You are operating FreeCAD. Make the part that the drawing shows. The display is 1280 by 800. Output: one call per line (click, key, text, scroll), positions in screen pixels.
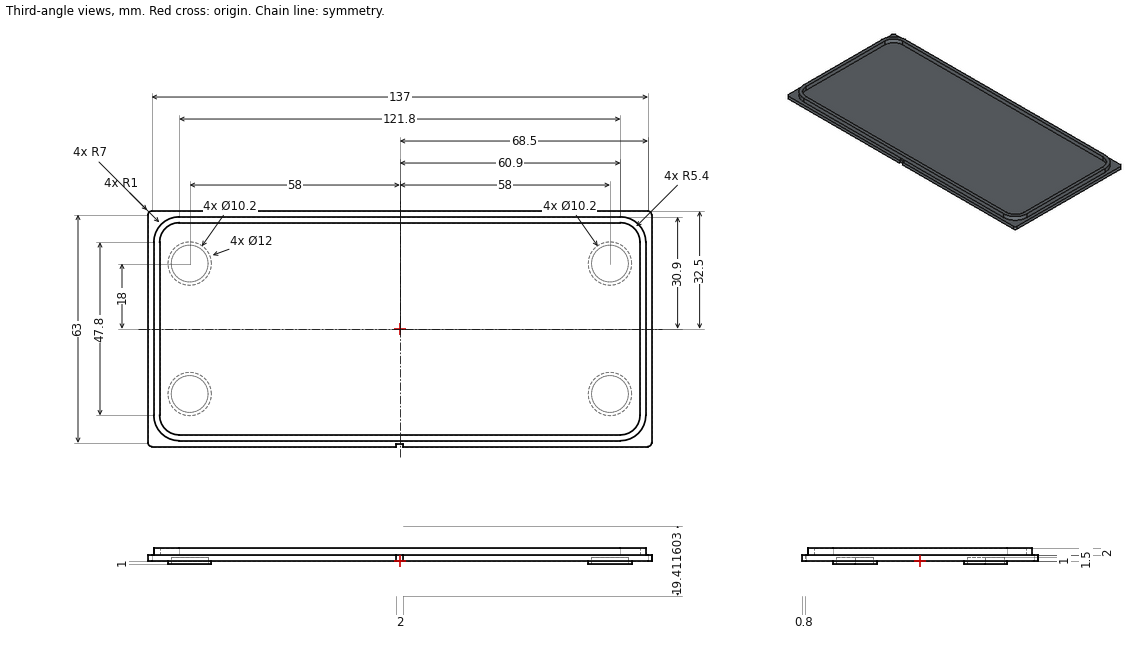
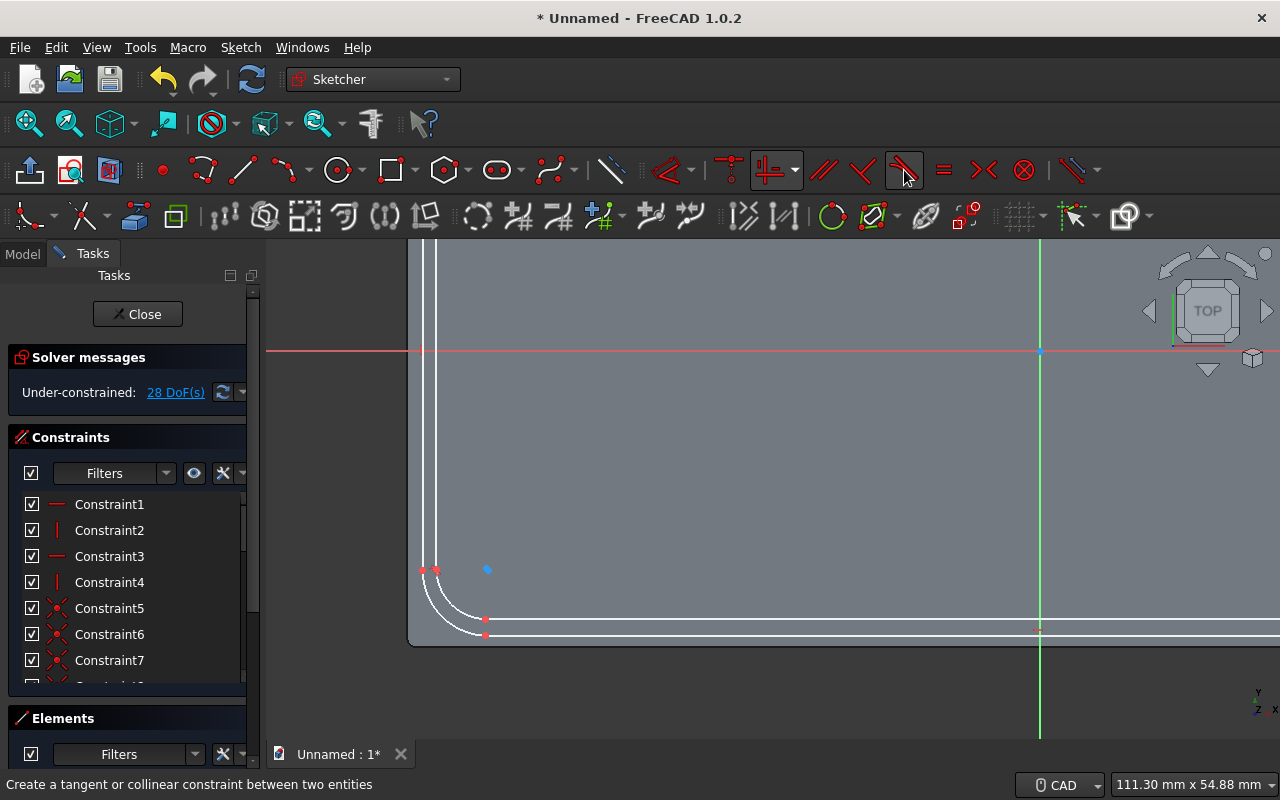
click(818, 636)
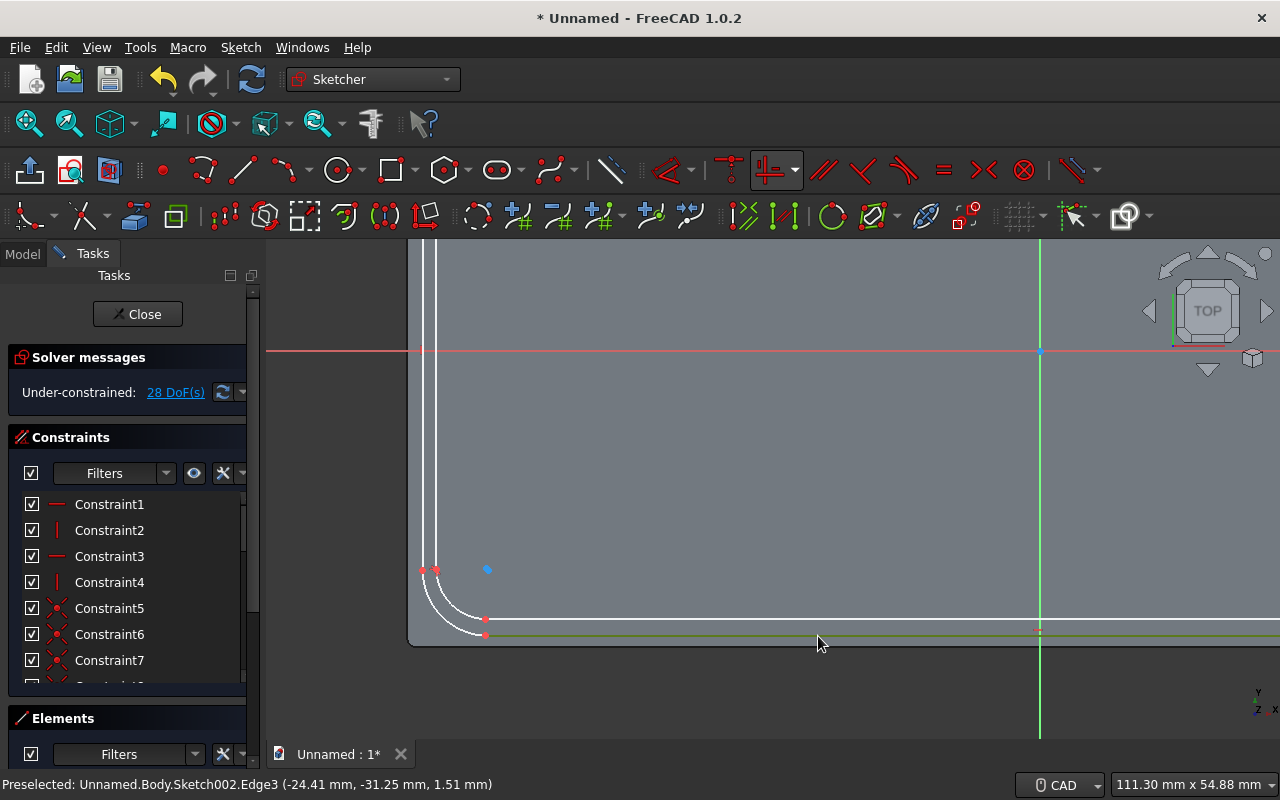
click(429, 599)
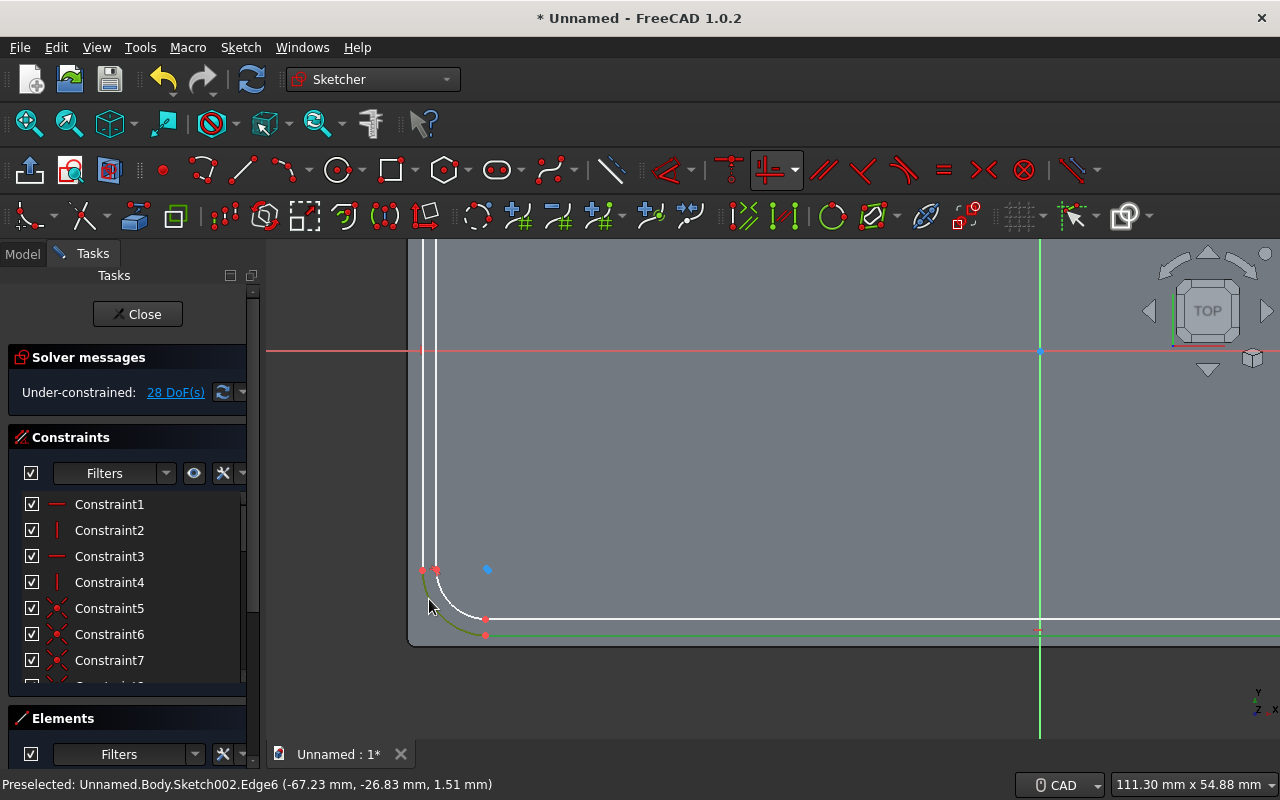
click(904, 170)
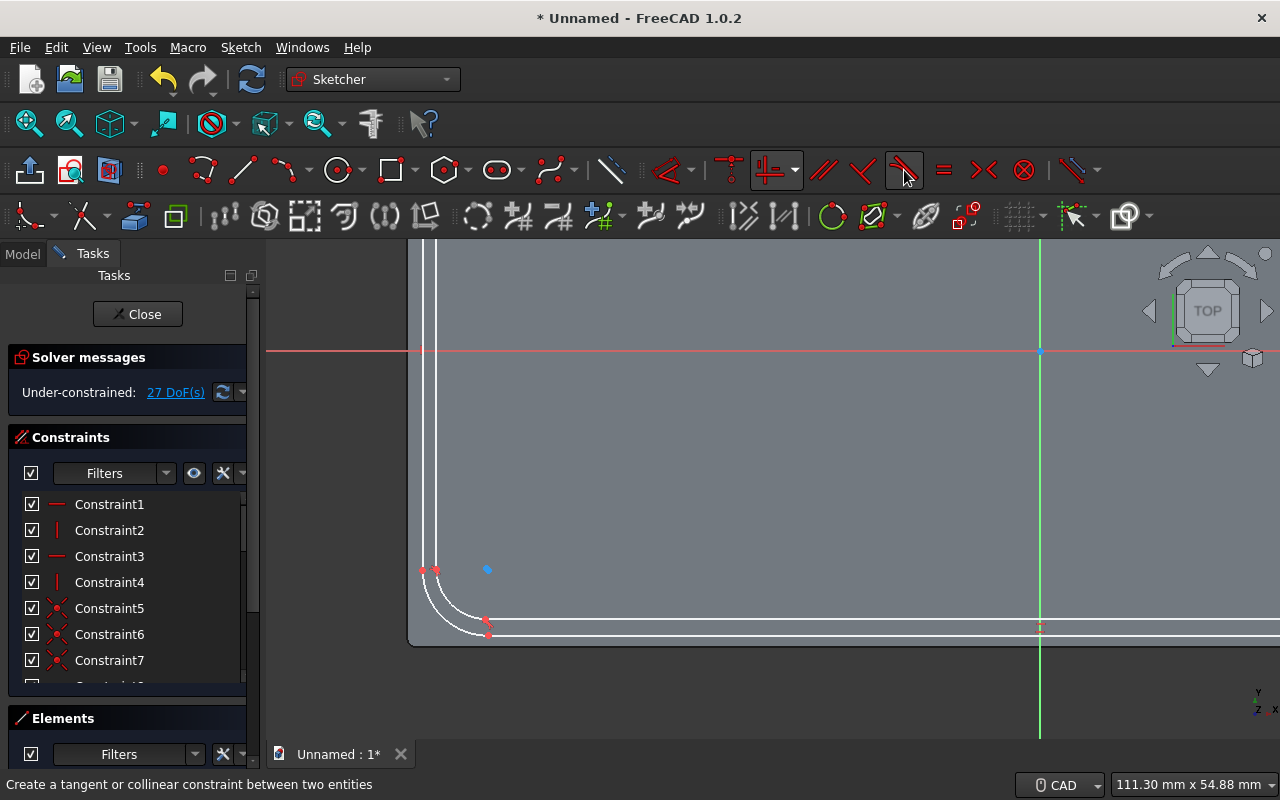
click(821, 636)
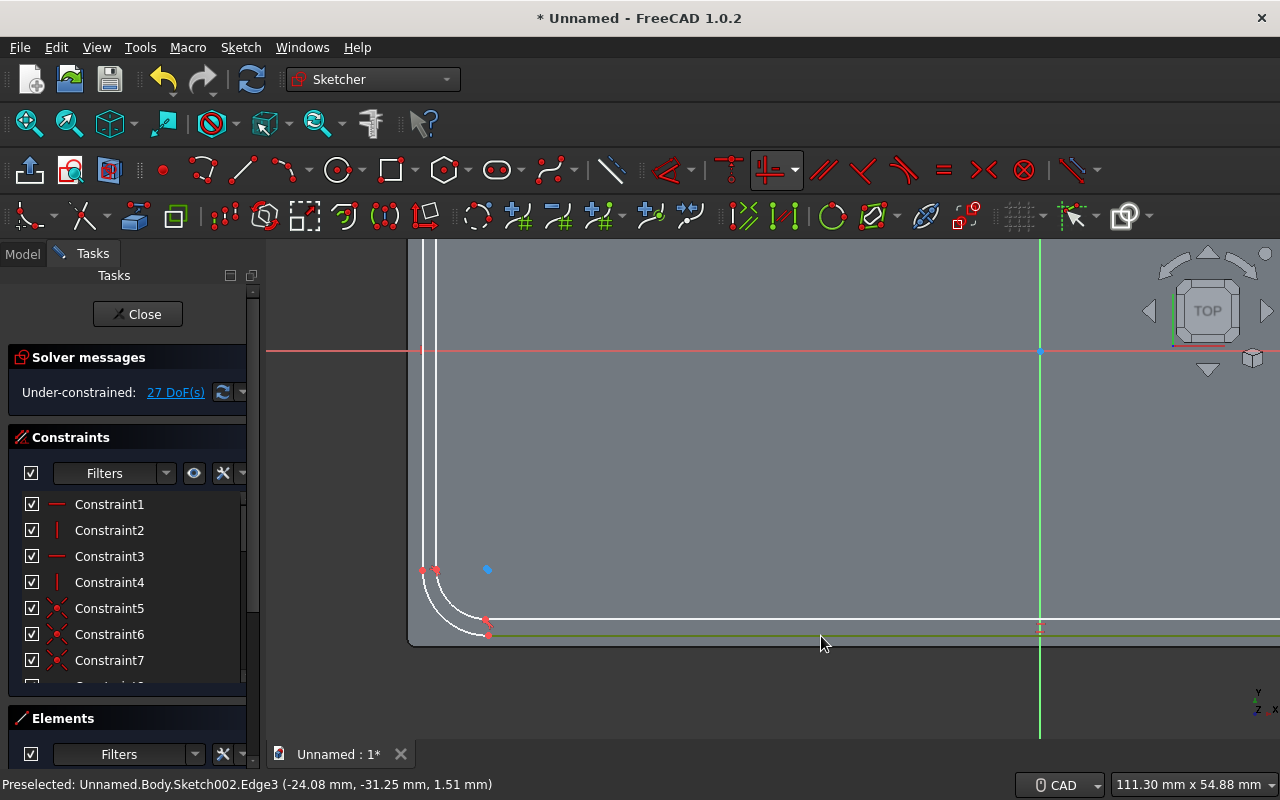
scroll(430, 602, down, 4)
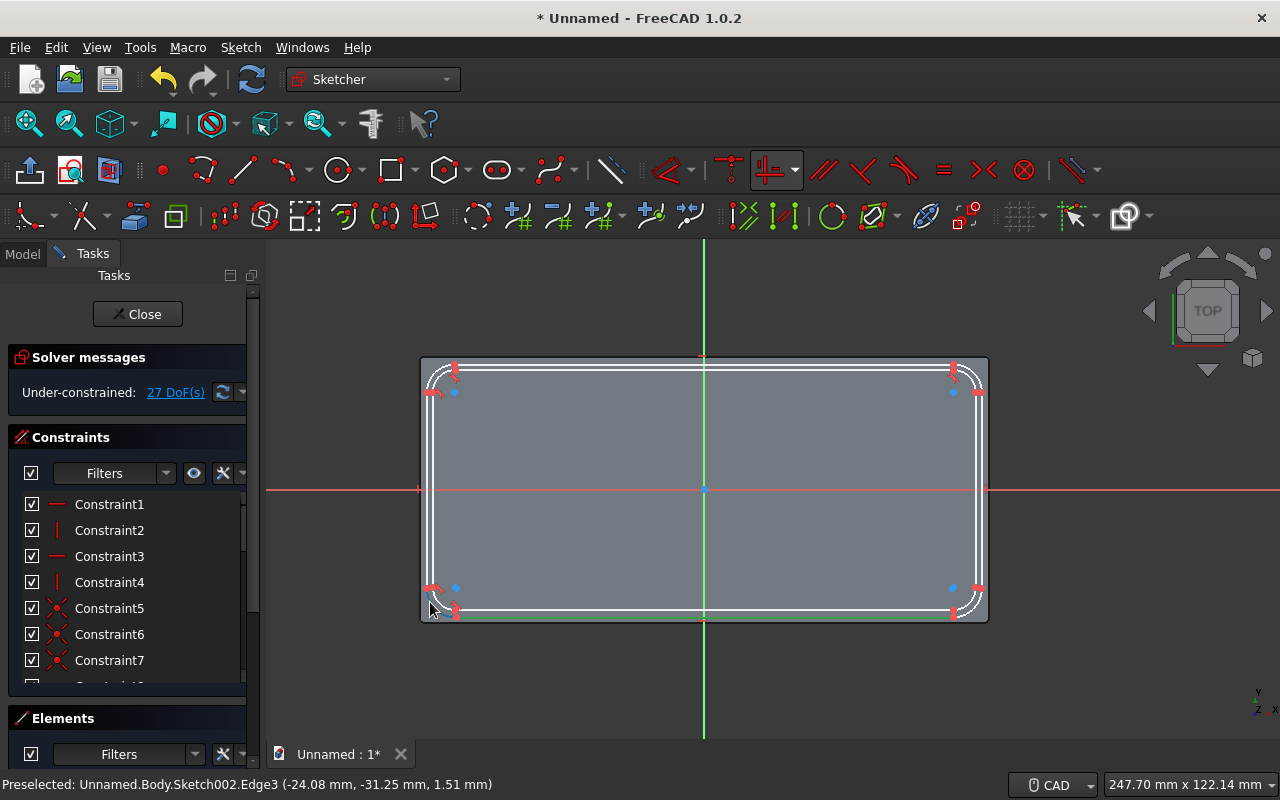
scroll(967, 614, up, 4)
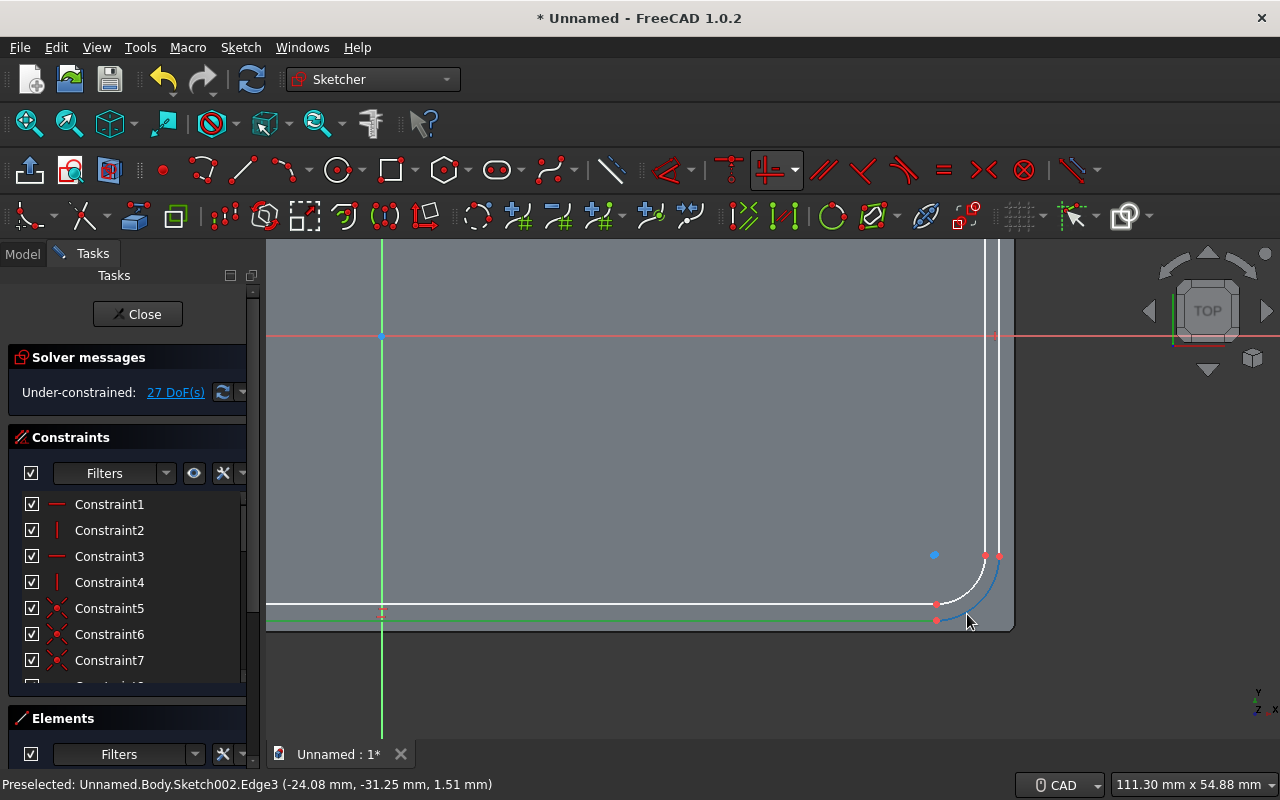
click(965, 613)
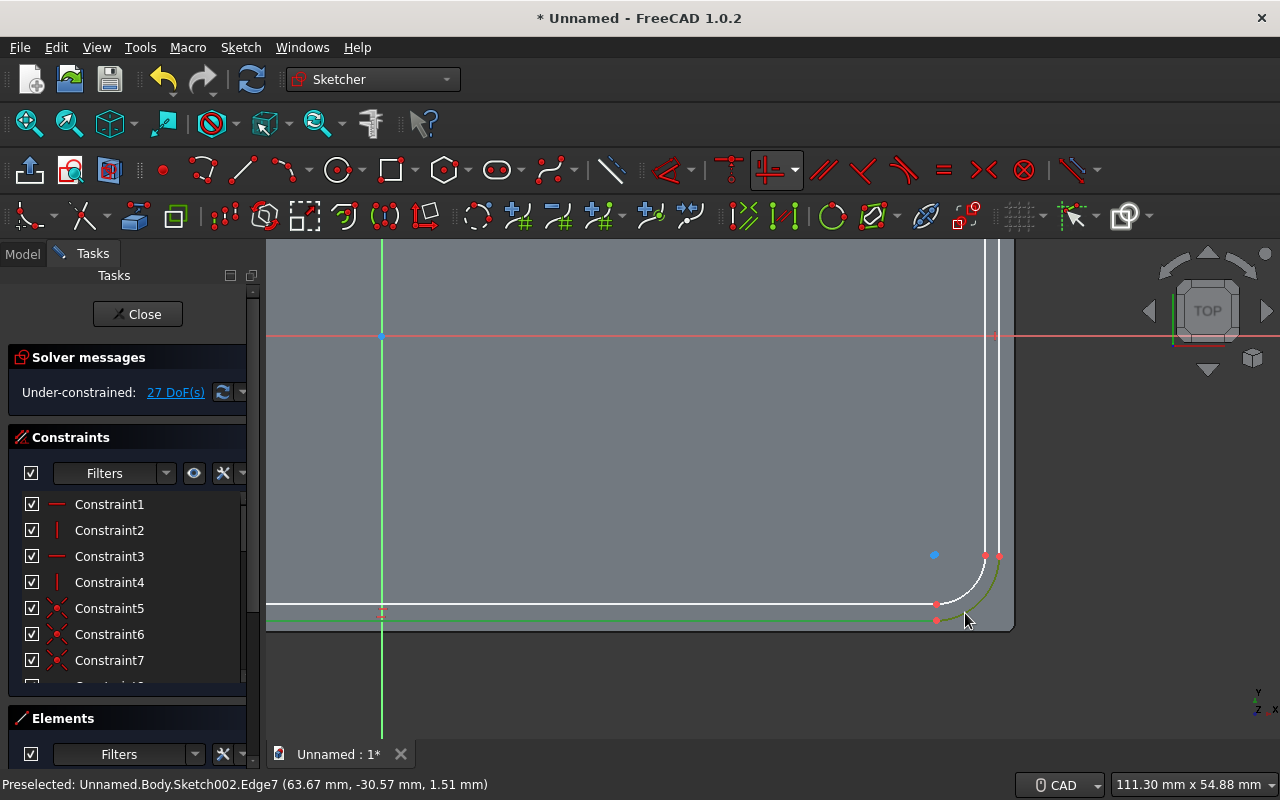
click(904, 170)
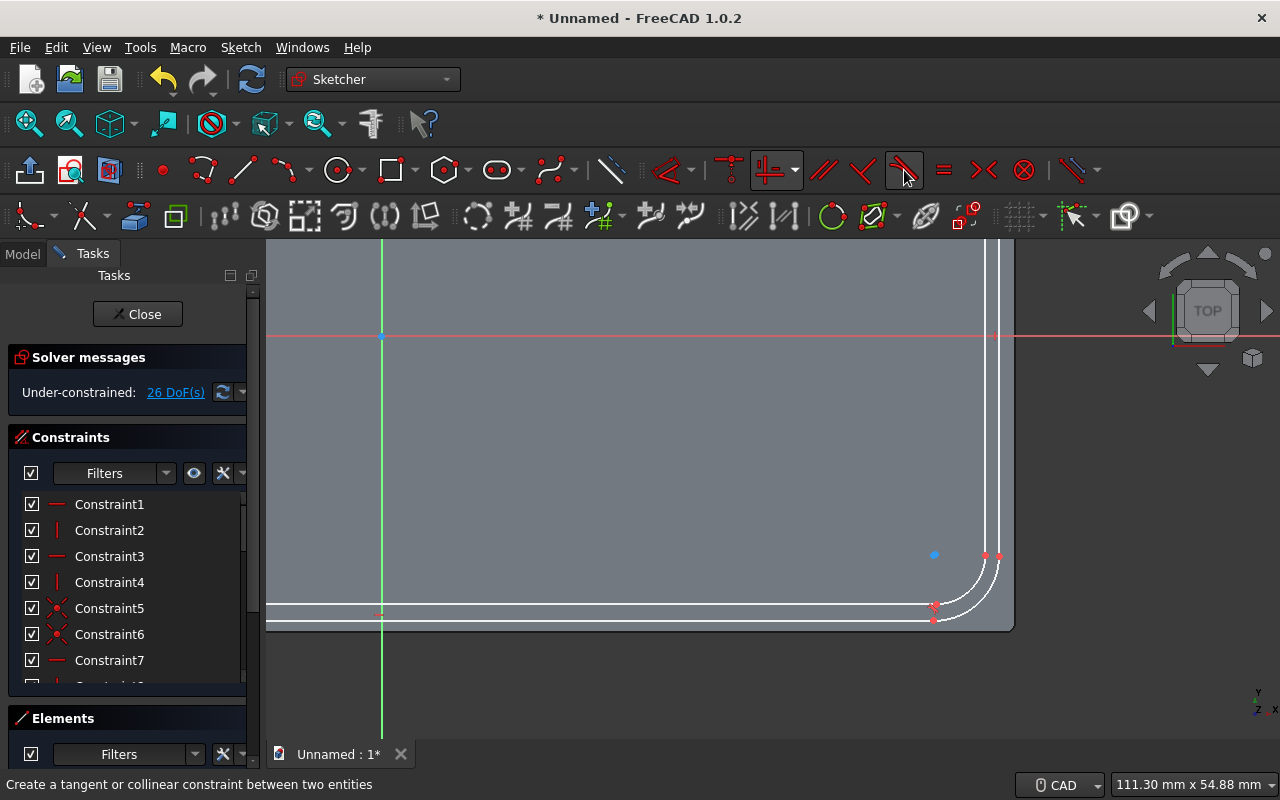
click(999, 426)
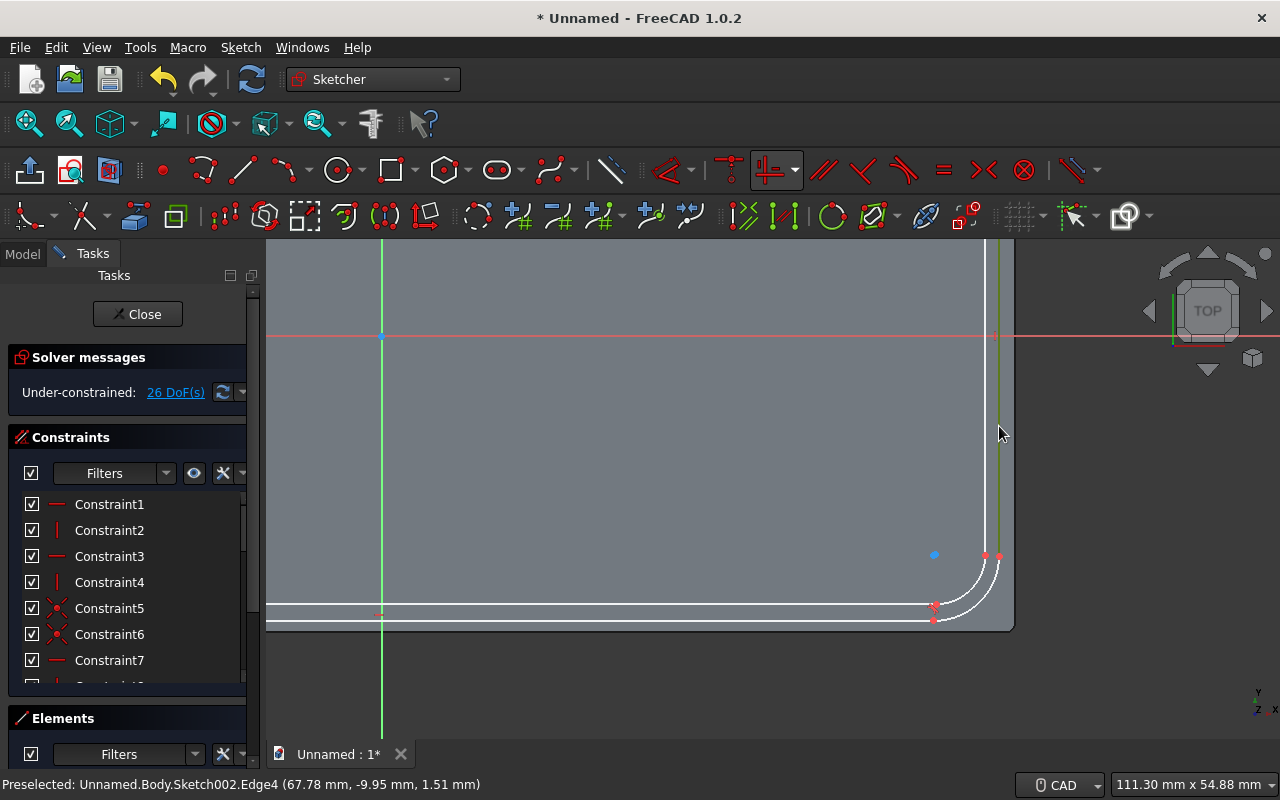
click(963, 614)